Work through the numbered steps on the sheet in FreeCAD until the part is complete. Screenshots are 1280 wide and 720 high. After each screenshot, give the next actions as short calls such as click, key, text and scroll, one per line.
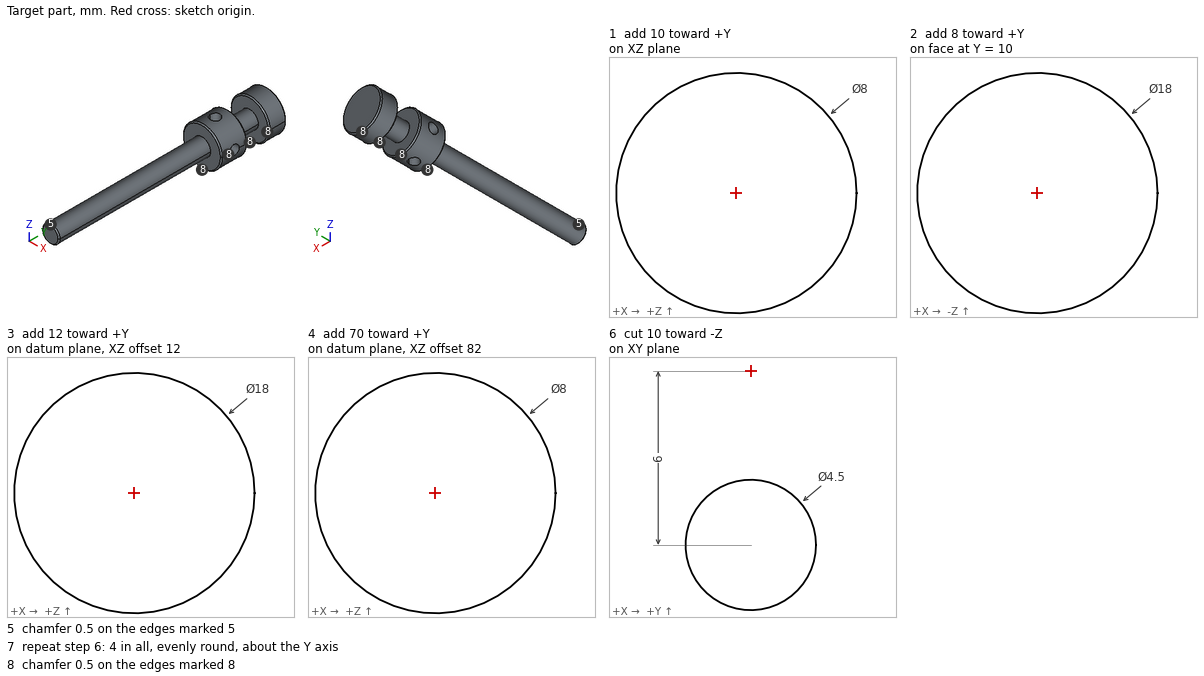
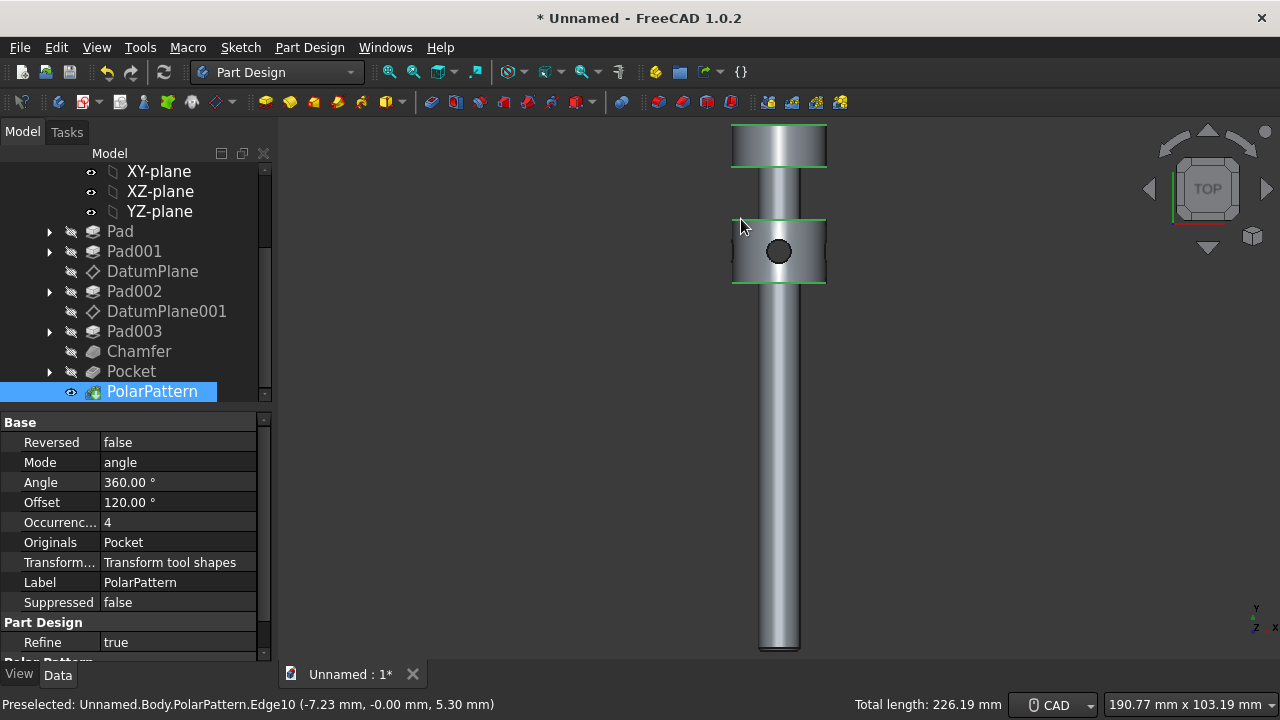
click(684, 102)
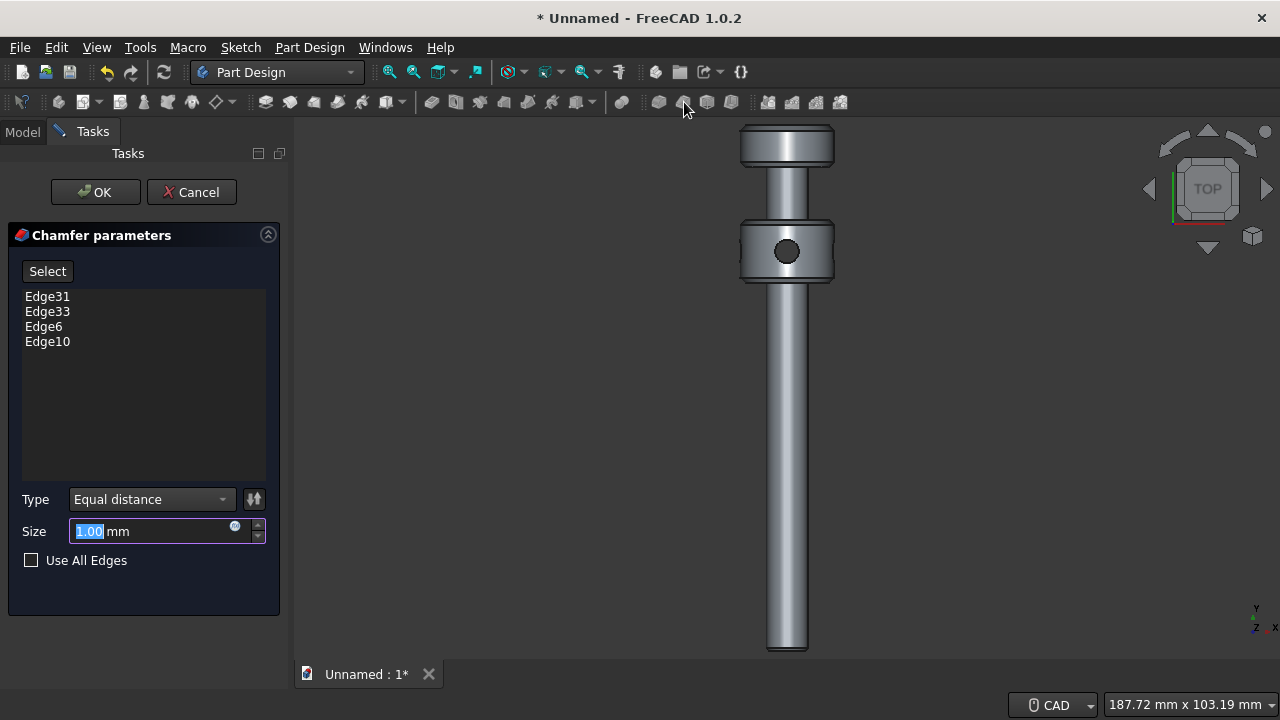
text(0.5)
key(Tab)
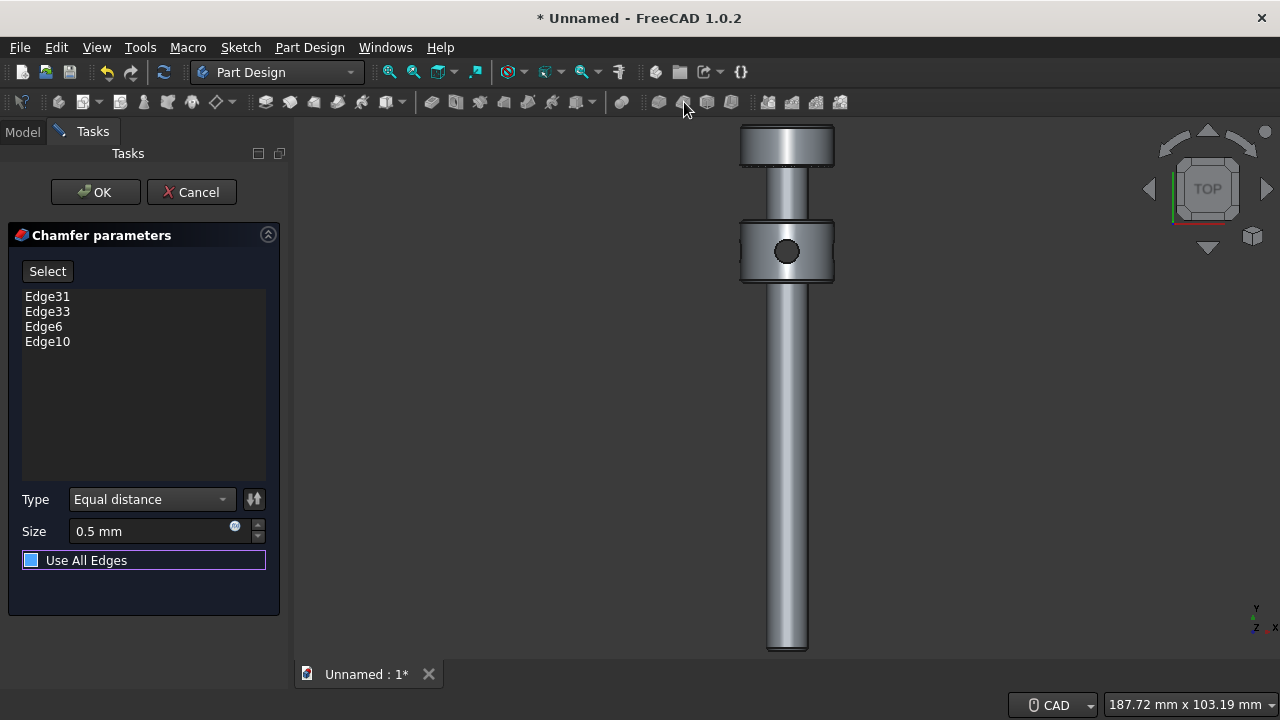
click(96, 192)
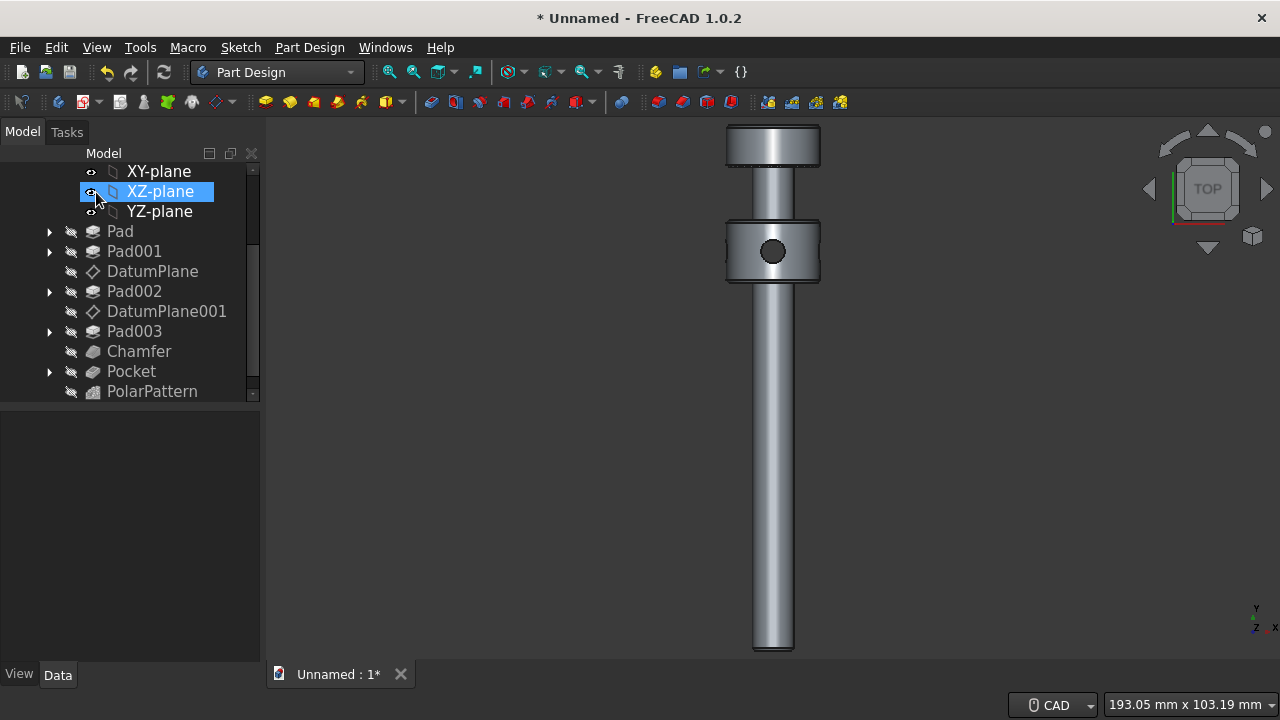
key(0)